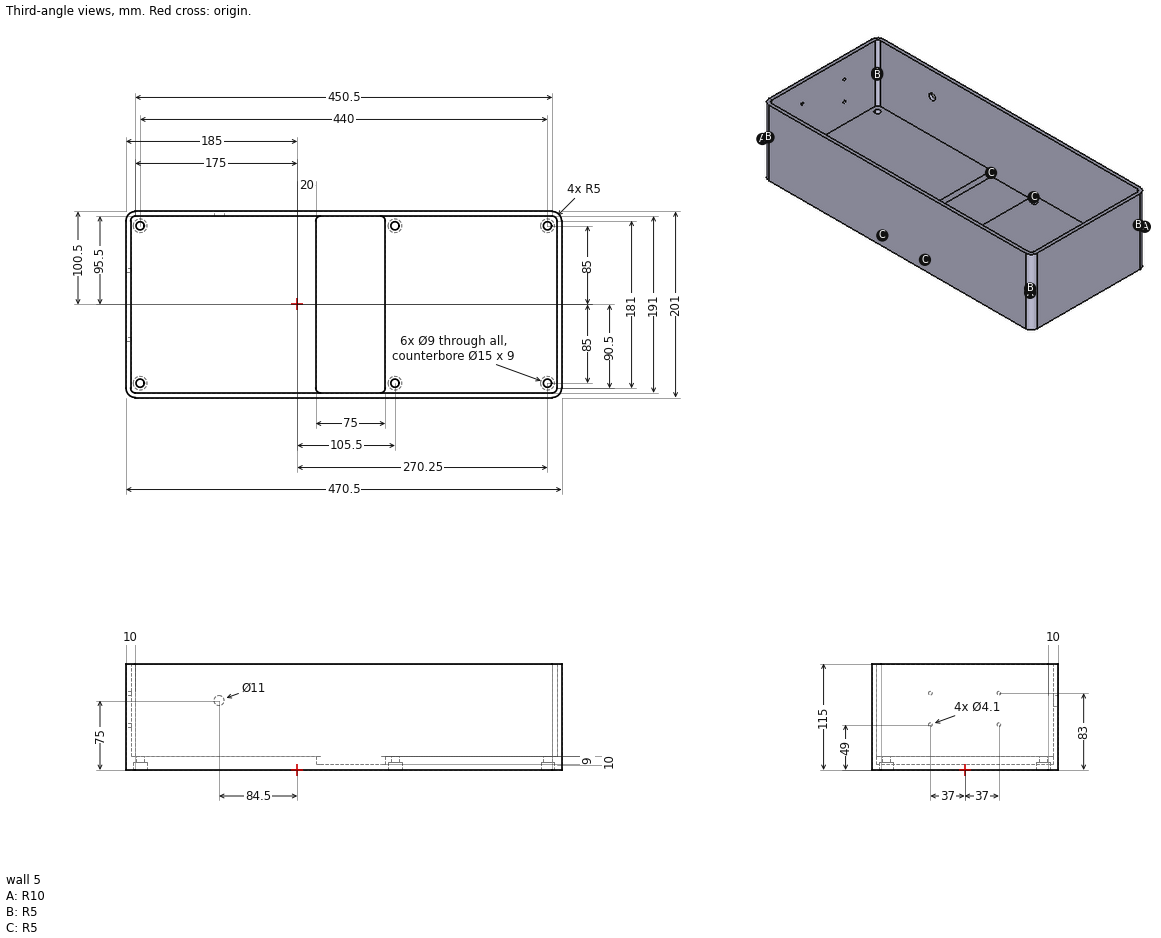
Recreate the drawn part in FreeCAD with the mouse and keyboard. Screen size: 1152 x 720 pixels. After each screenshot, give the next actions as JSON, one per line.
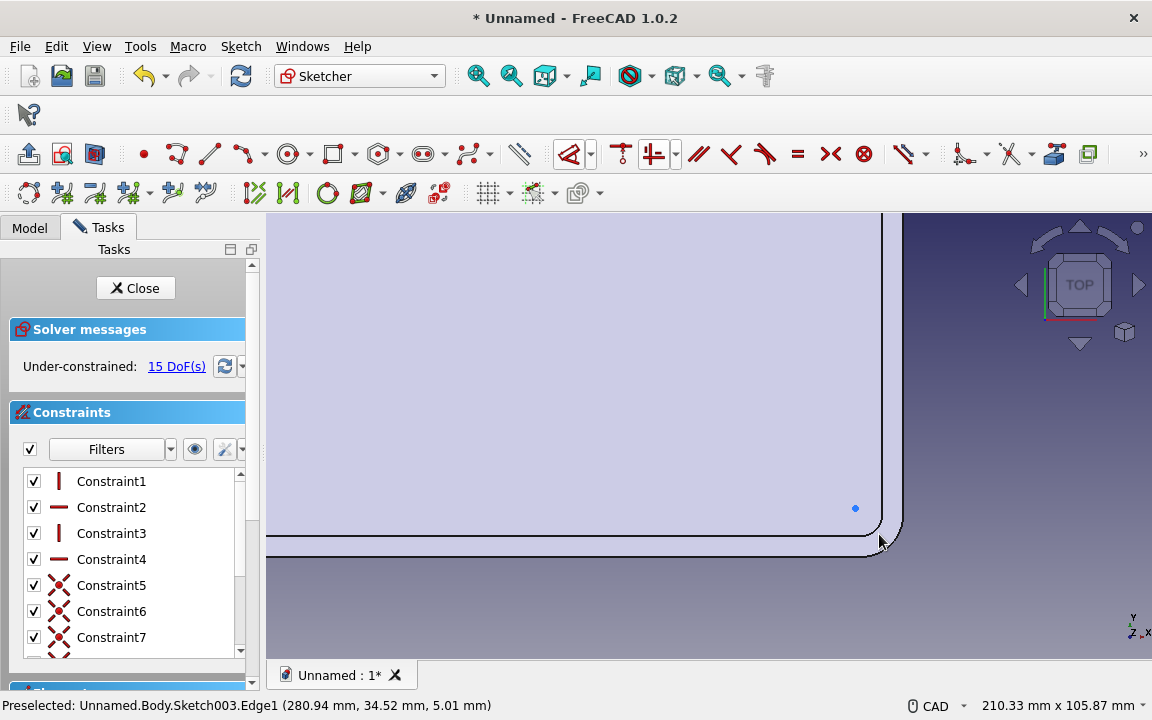
{"action": "left_click", "coordinate": [875, 532]}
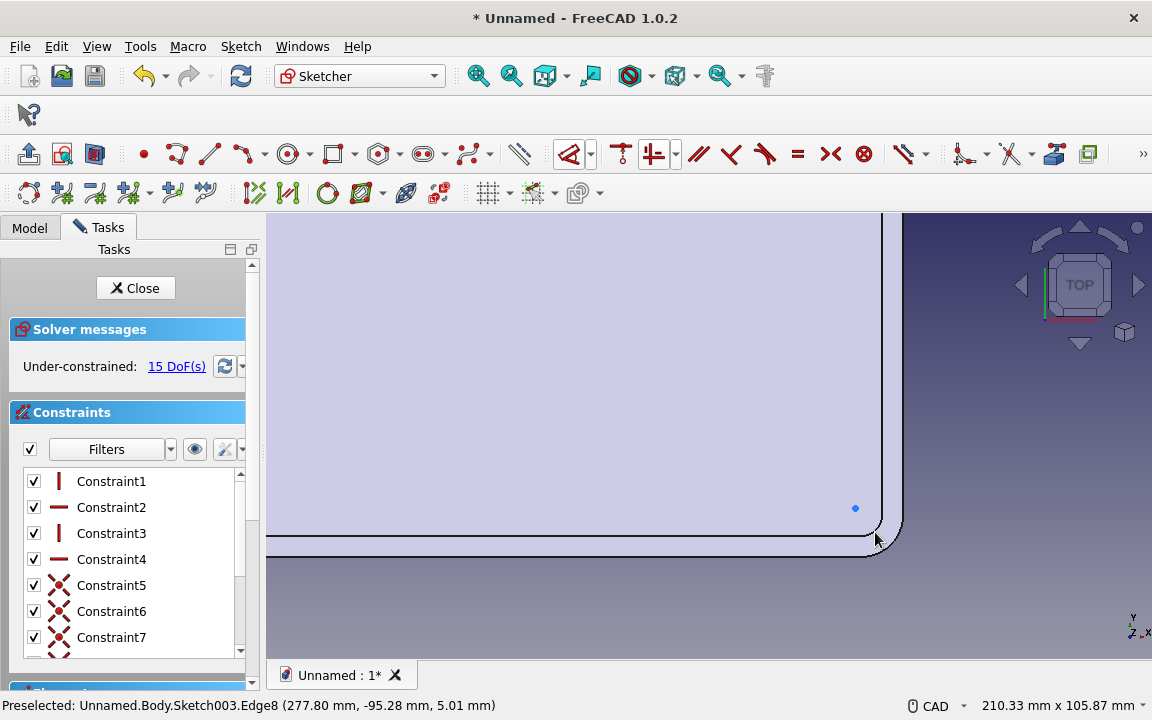
{"action": "key", "text": "t"}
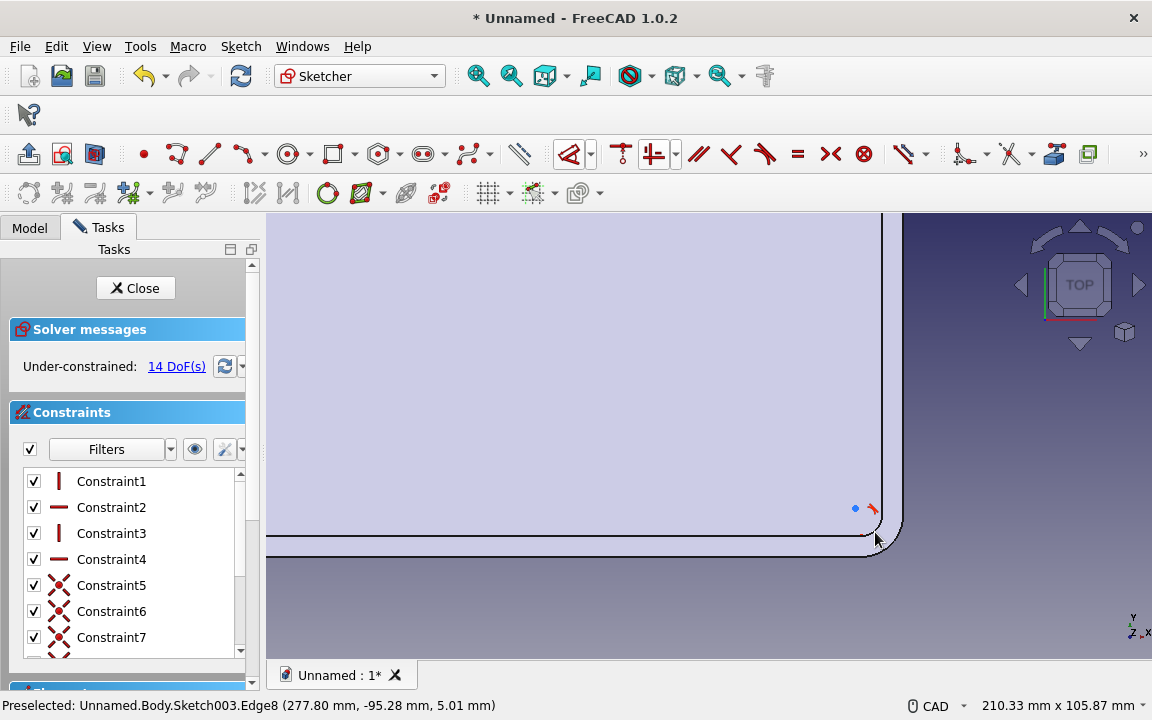
{"action": "scroll", "coordinate": [879, 535], "scroll_direction": "down", "scroll_amount": 7}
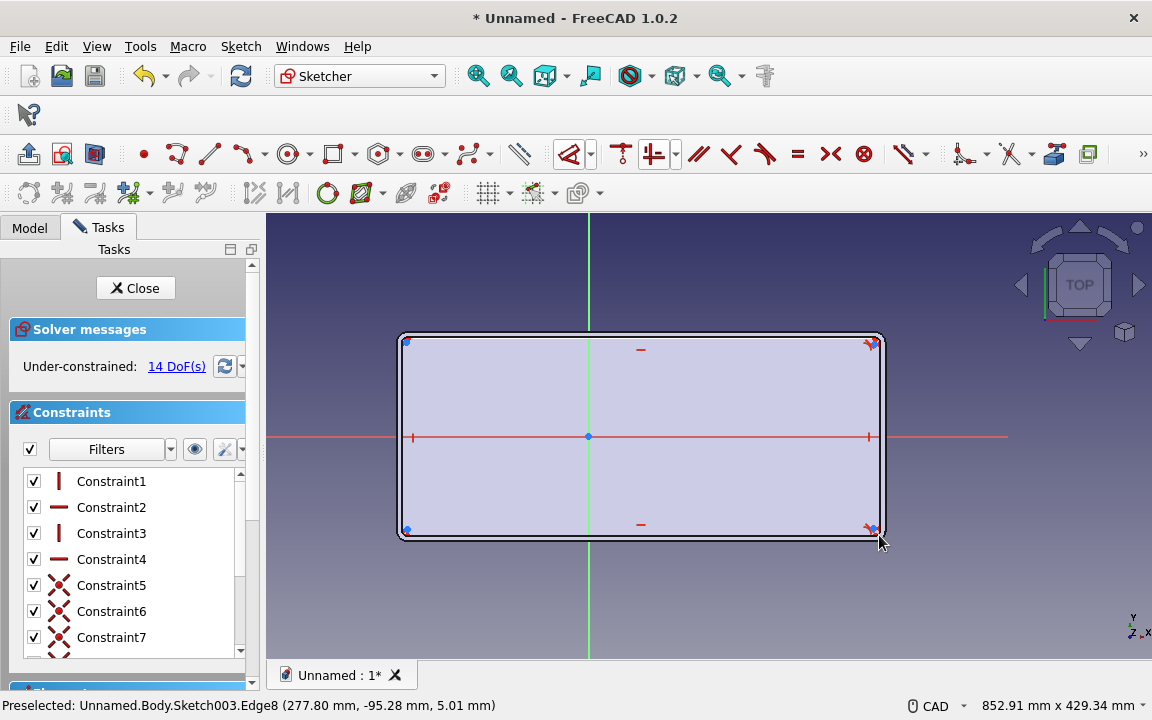
{"action": "left_click", "coordinate": [735, 338]}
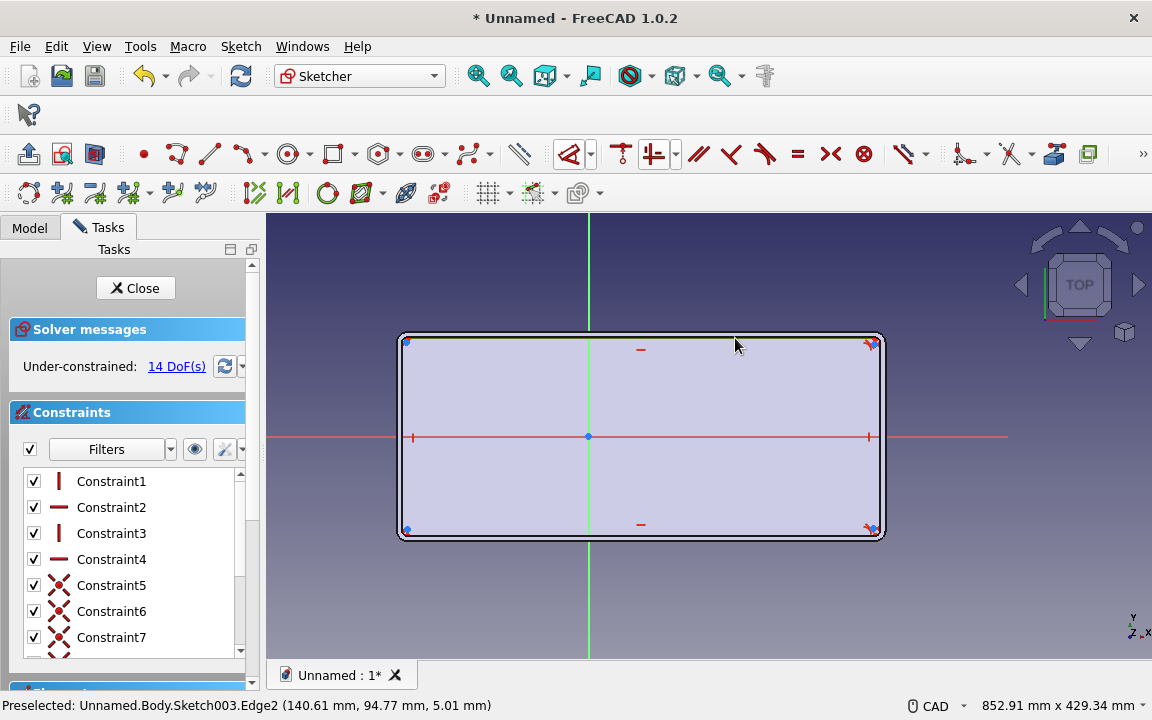
{"action": "scroll", "coordinate": [879, 340], "scroll_direction": "up", "scroll_amount": 6}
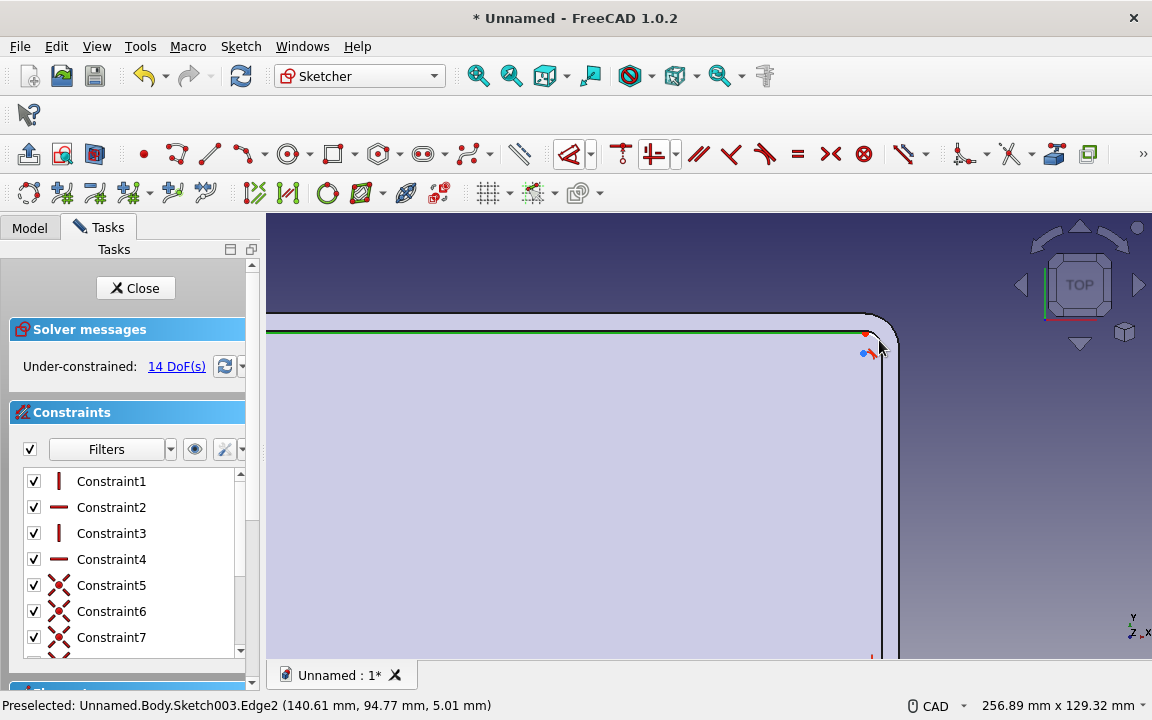
{"action": "left_click", "coordinate": [878, 340]}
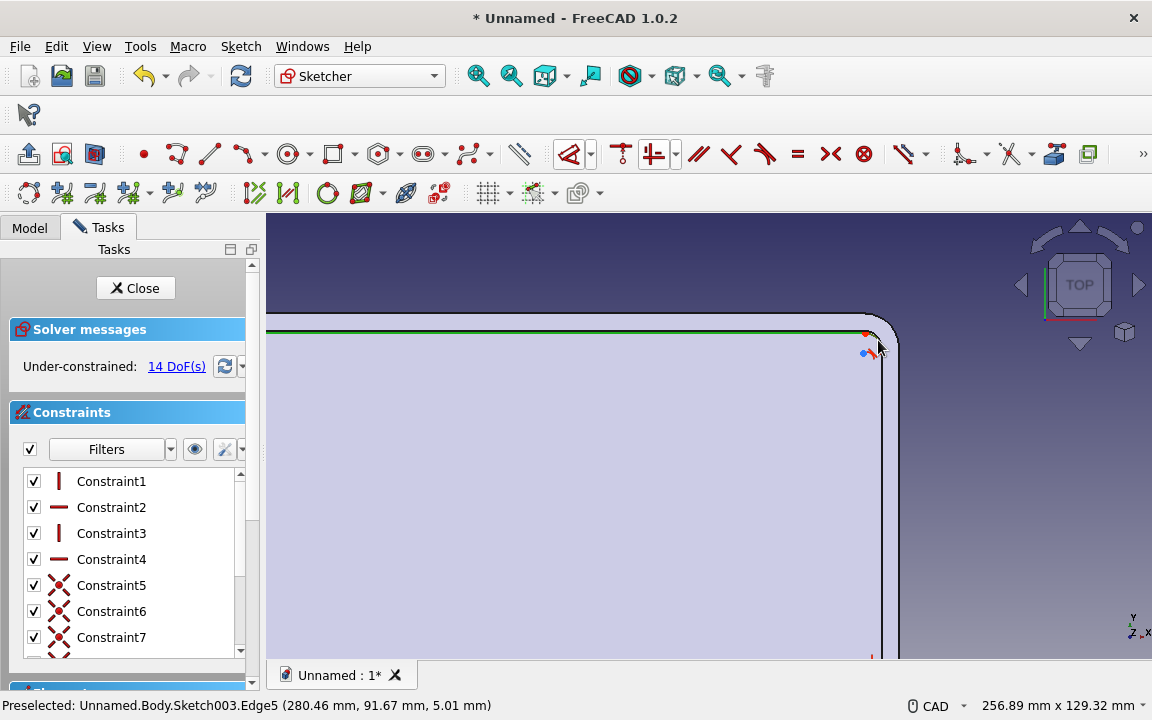
{"action": "key", "text": "t"}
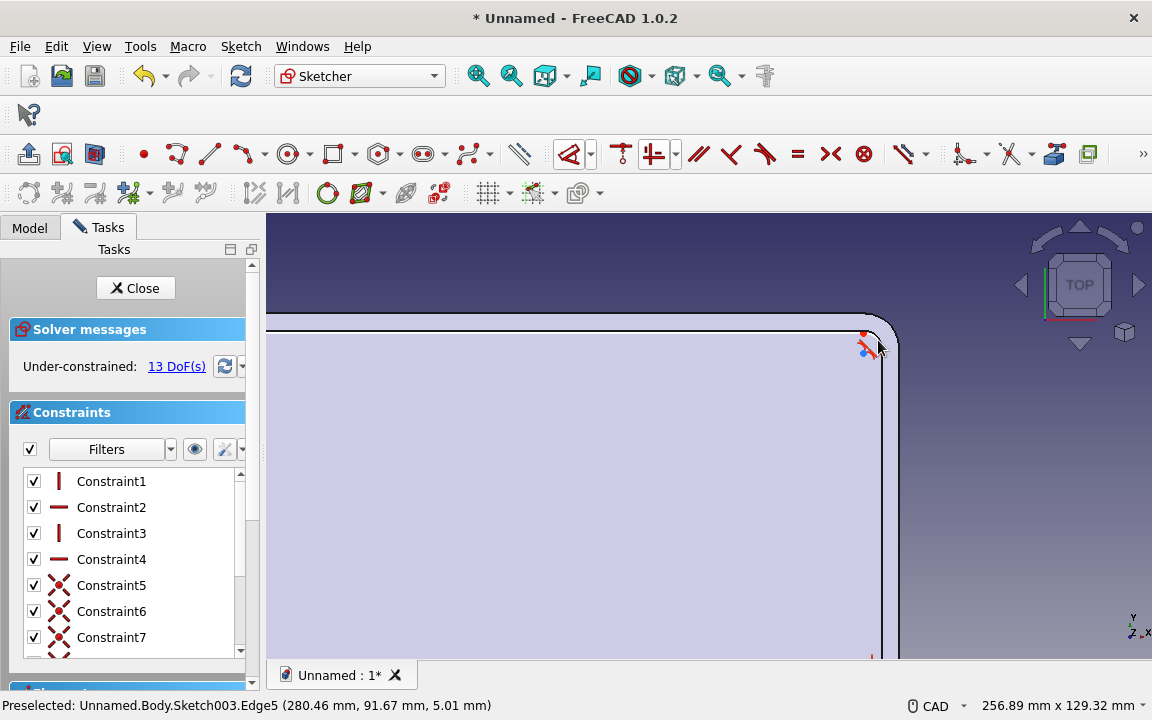
{"action": "scroll", "coordinate": [879, 339], "scroll_direction": "down", "scroll_amount": 6}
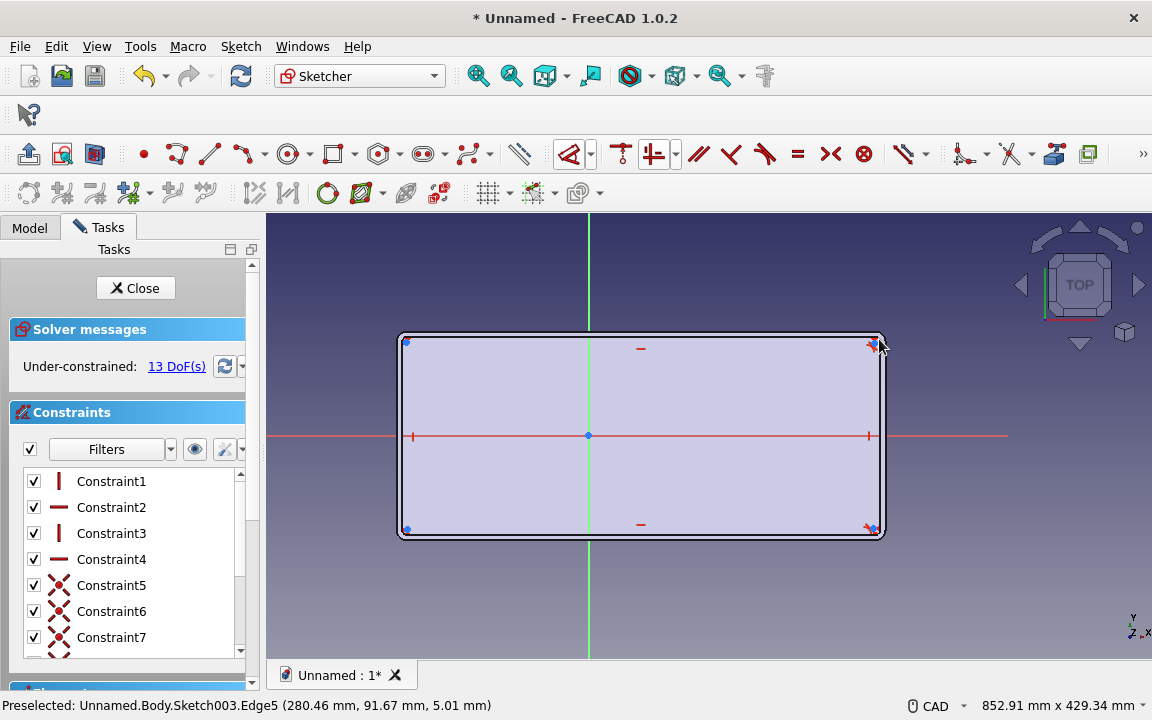
{"action": "left_click", "coordinate": [735, 337]}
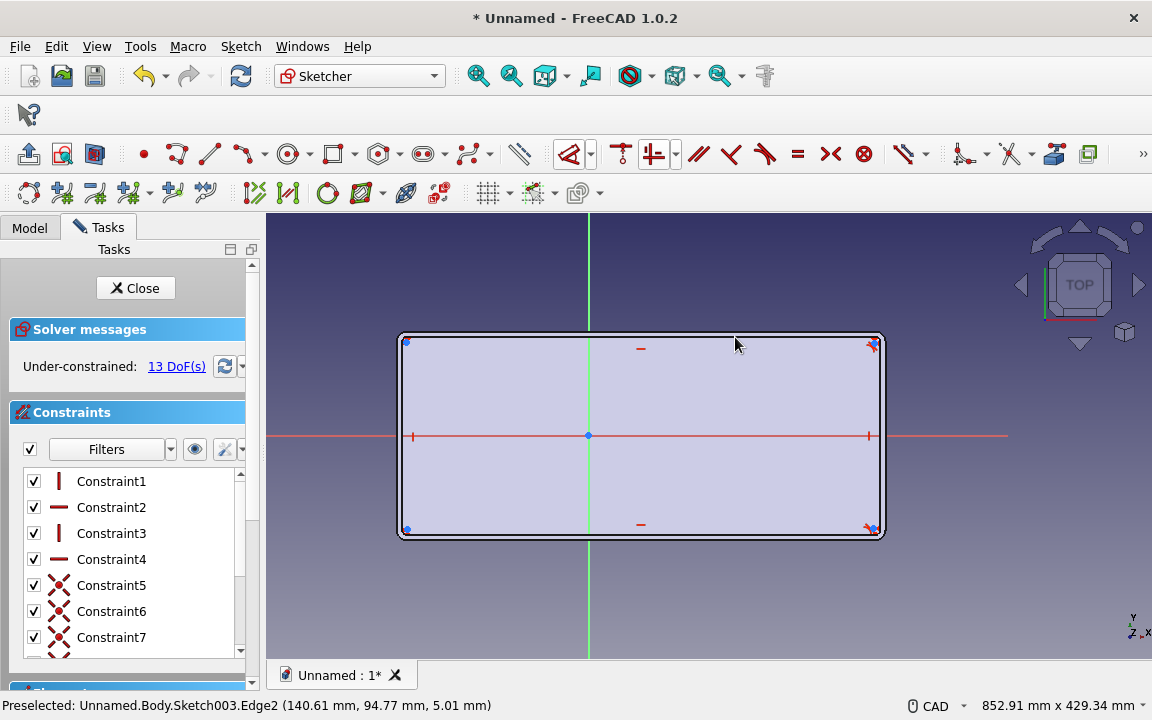
{"action": "scroll", "coordinate": [403, 339], "scroll_direction": "up", "scroll_amount": 7}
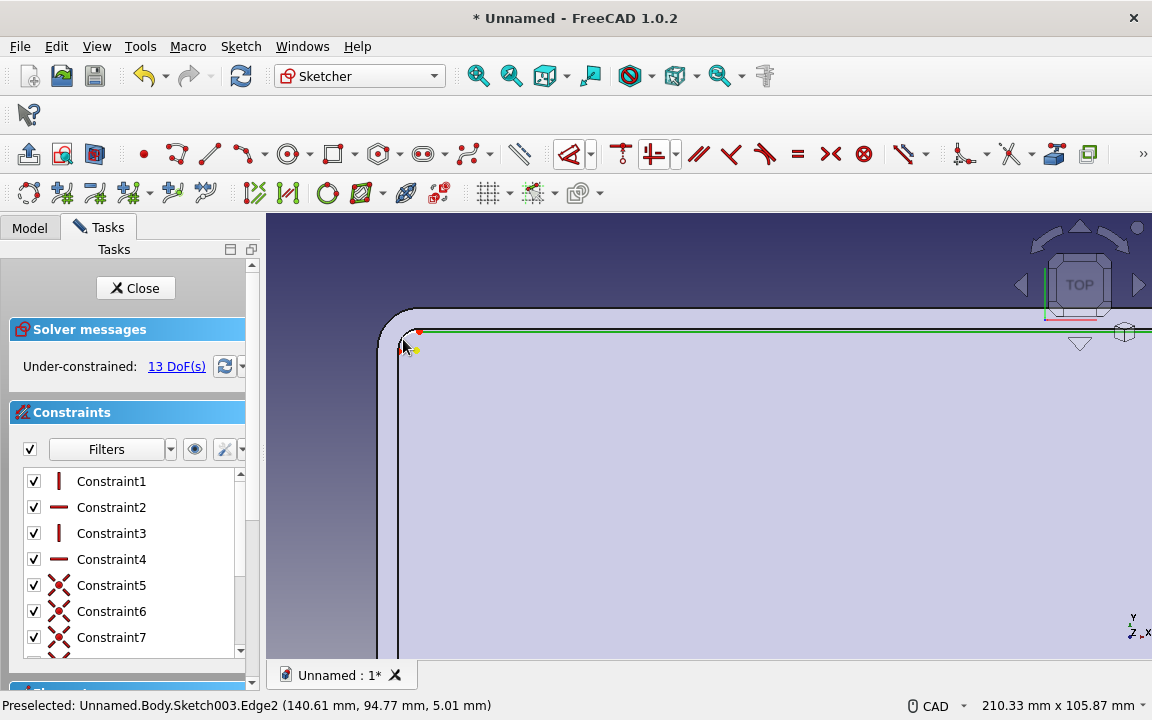
{"action": "left_click", "coordinate": [404, 337]}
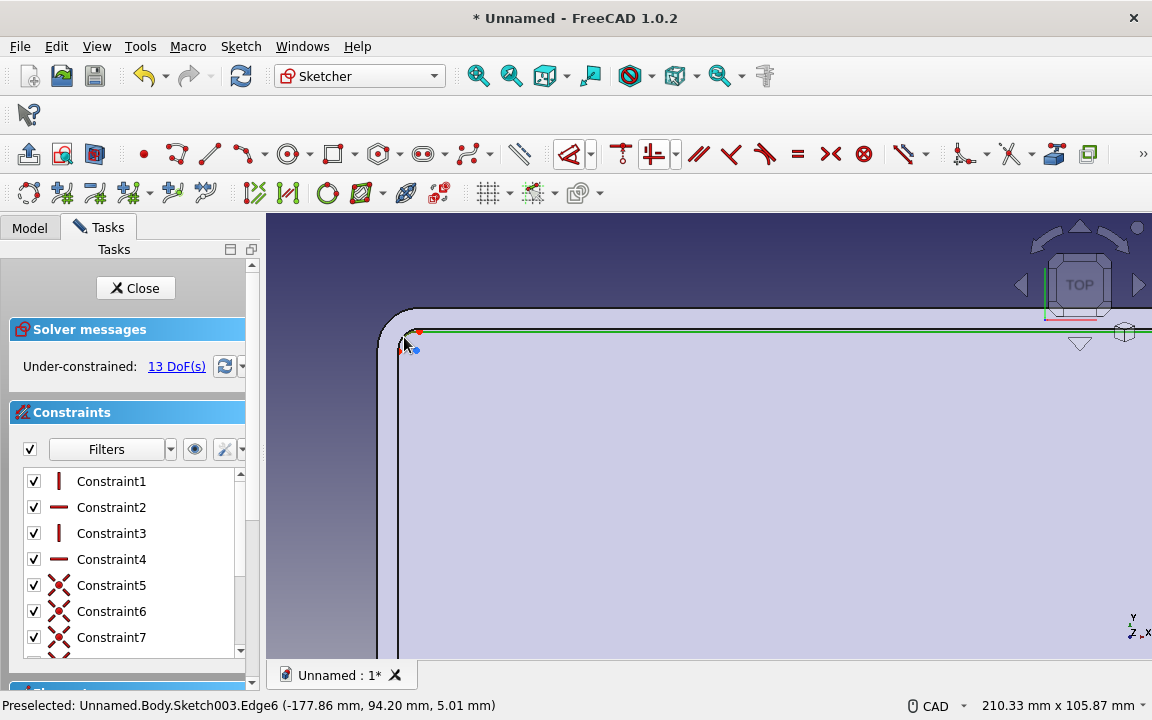
{"action": "key", "text": "t"}